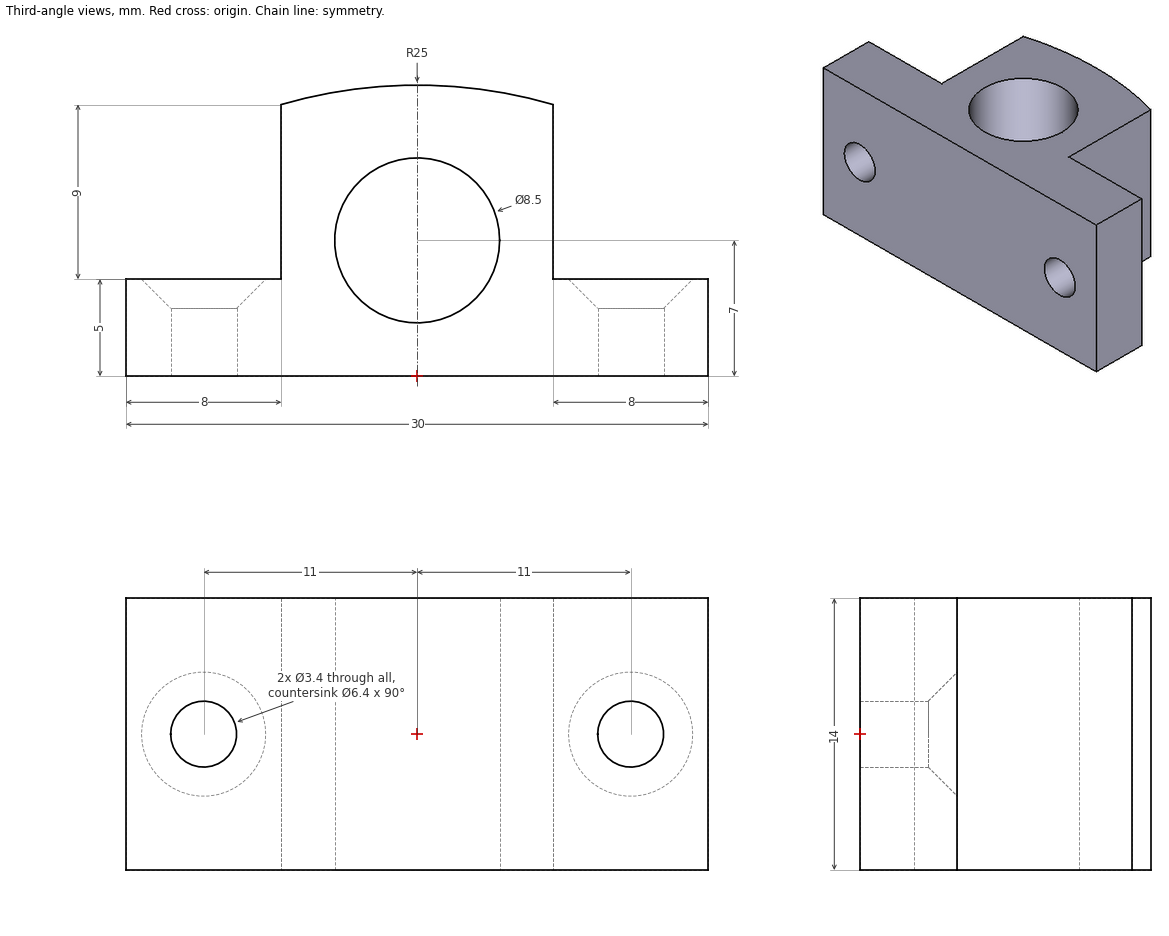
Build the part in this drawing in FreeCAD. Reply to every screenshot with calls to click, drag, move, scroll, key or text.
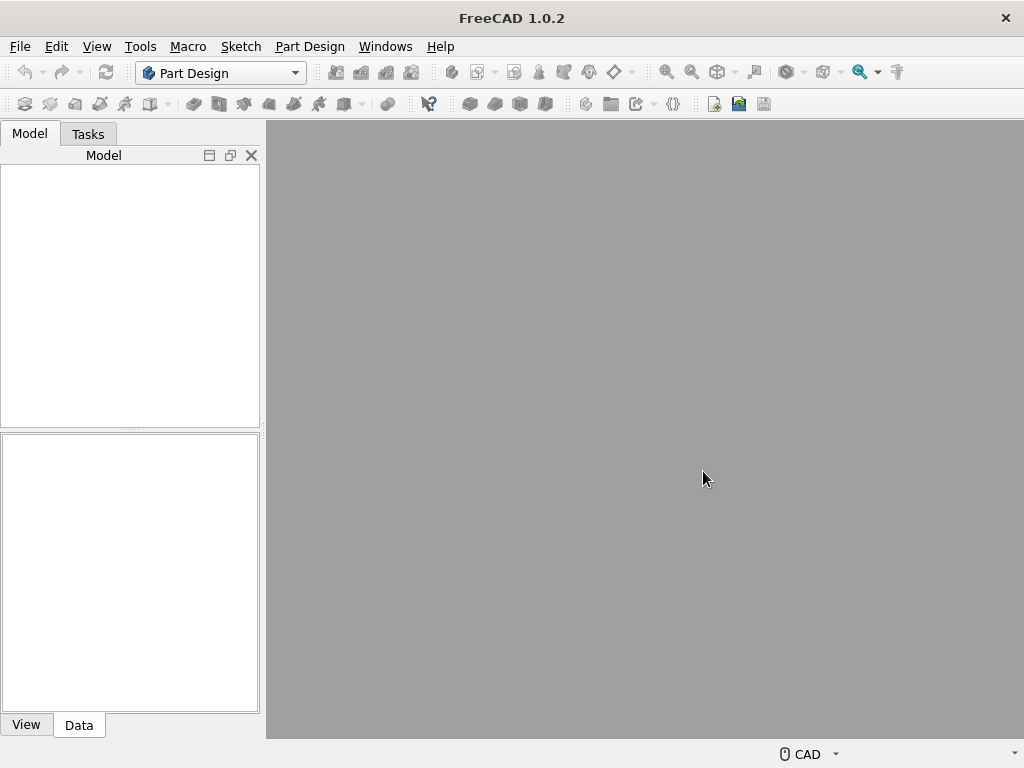
click(714, 104)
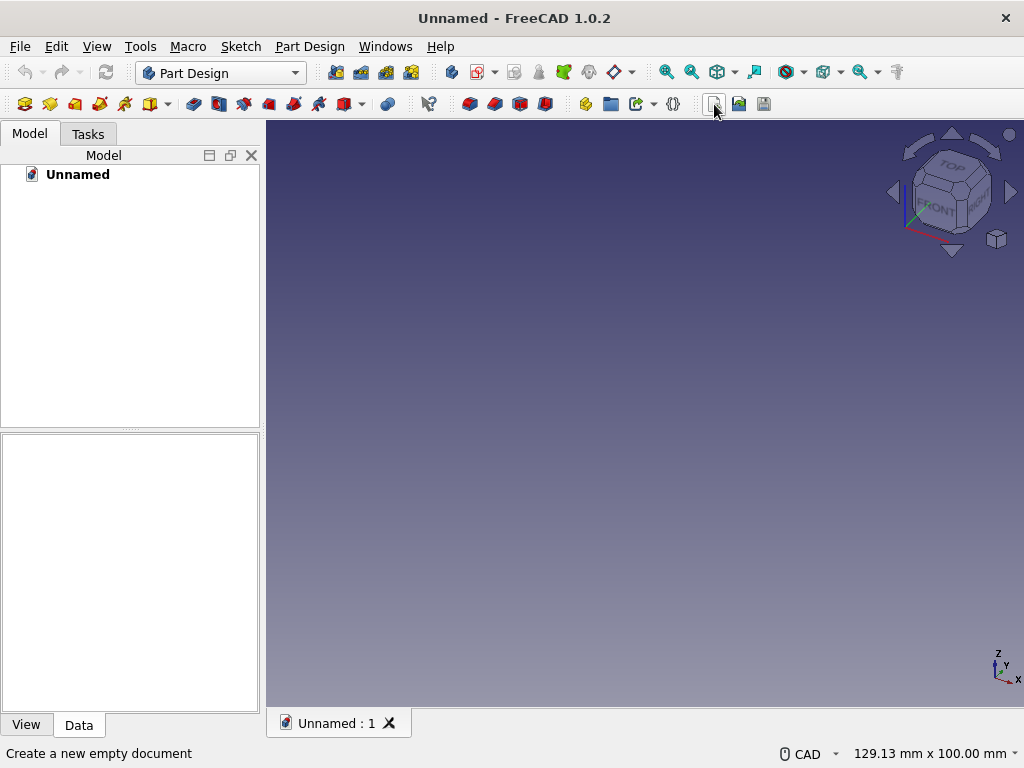
click(476, 72)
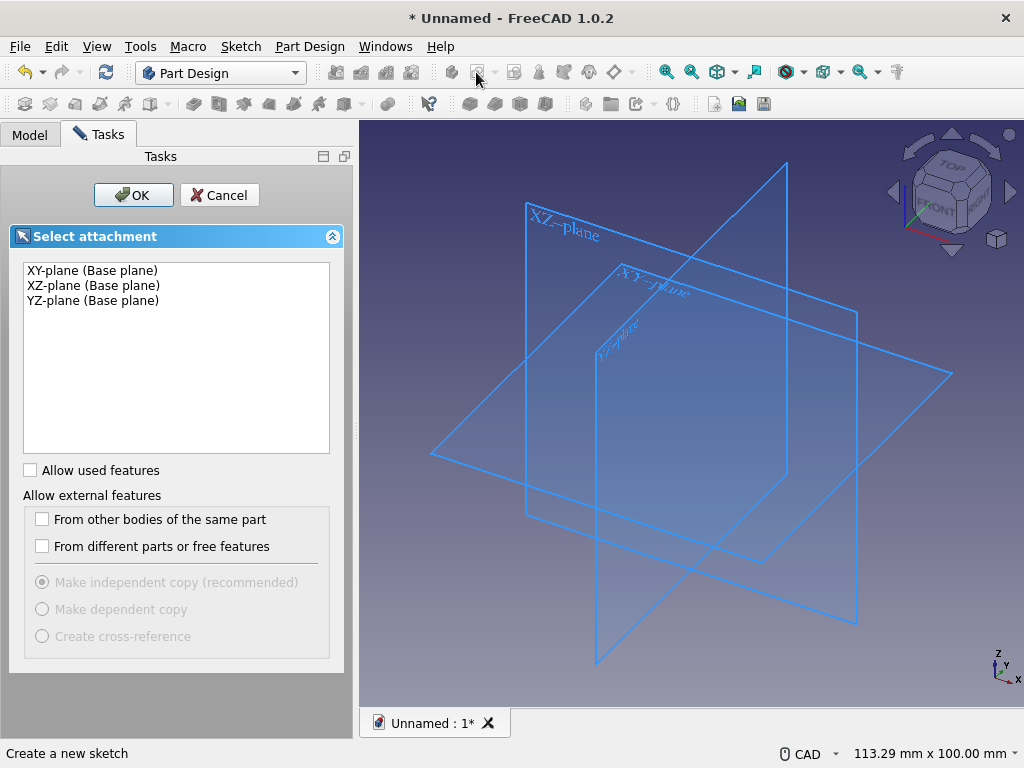
click(84, 270)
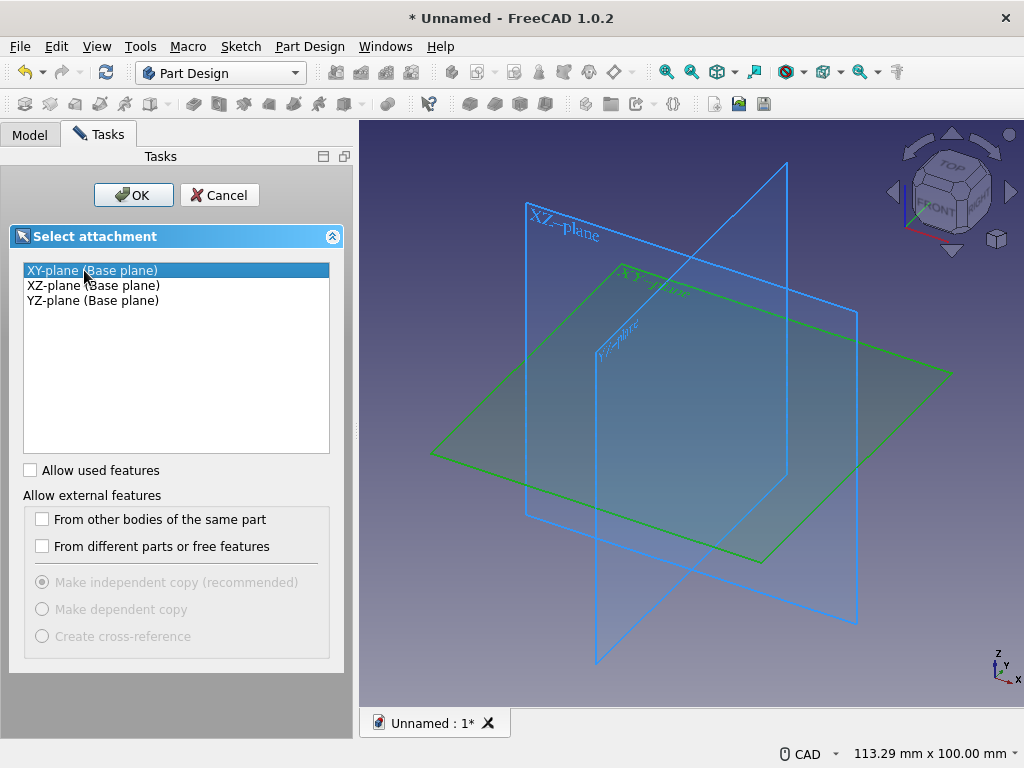
click(134, 195)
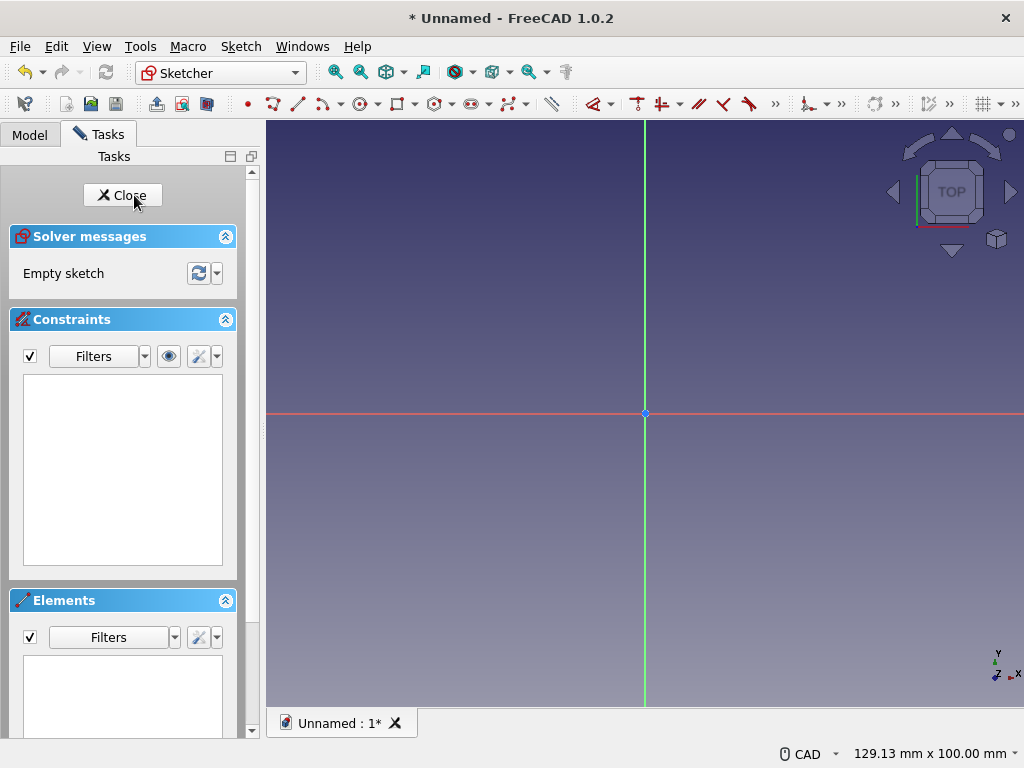
scroll(701, 334, up, 4)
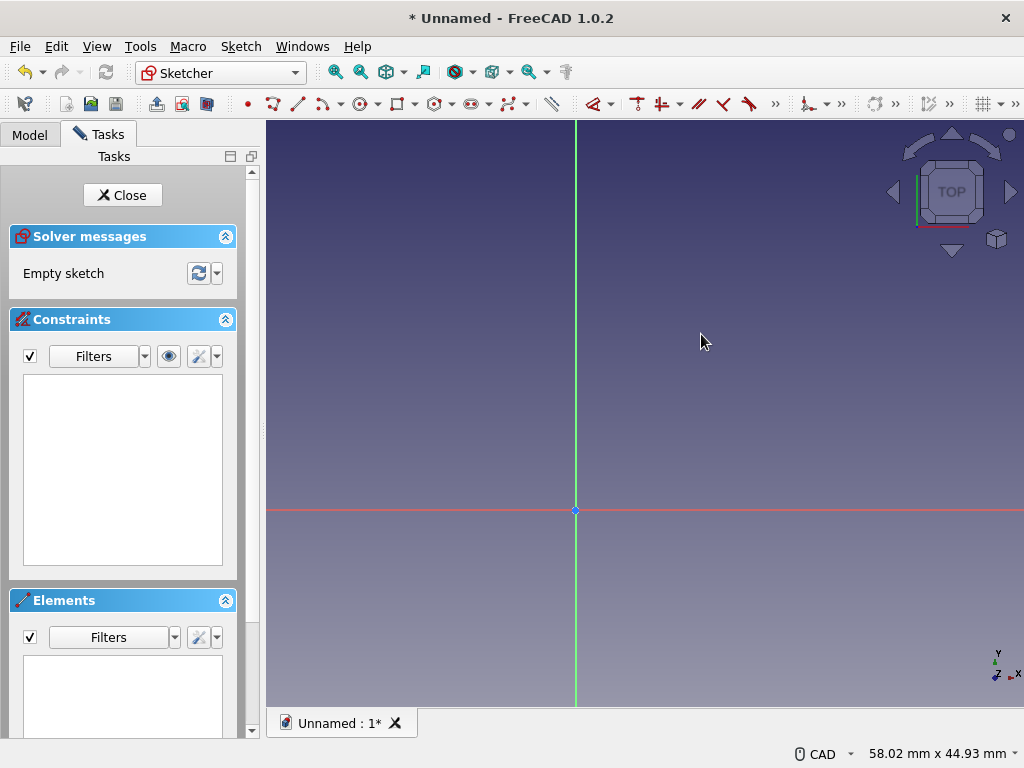
click(273, 104)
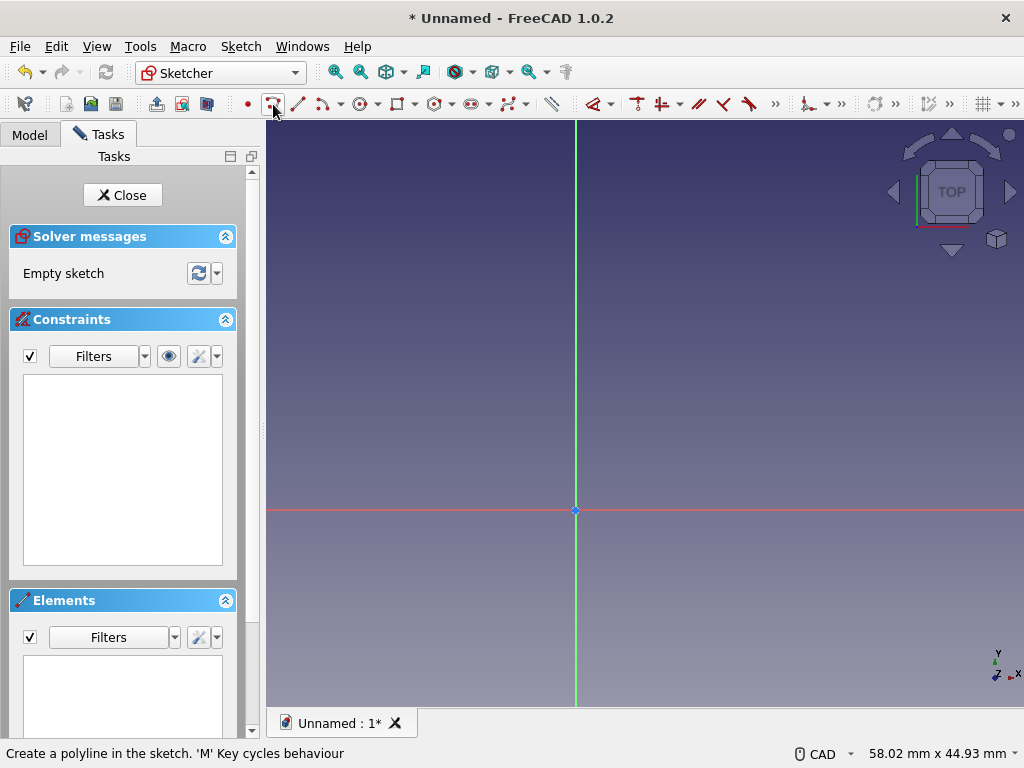
click(484, 328)
click(484, 445)
click(380, 445)
click(380, 510)
click(772, 501)
click(772, 445)
click(667, 445)
click(667, 328)
right_click(667, 328)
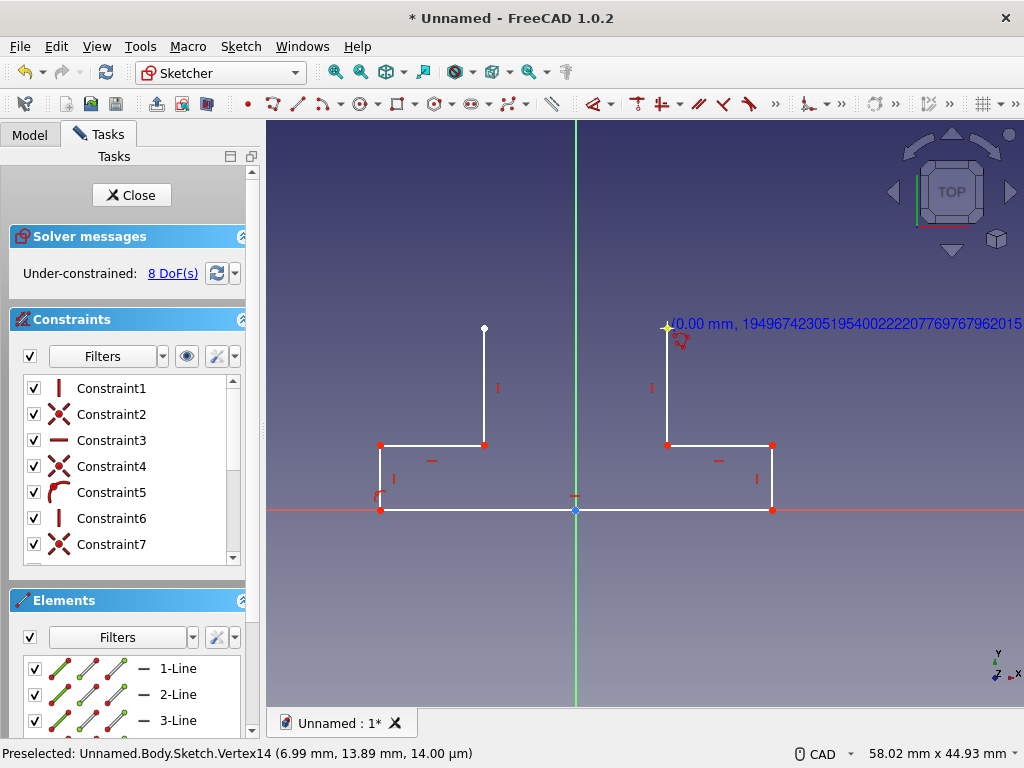
click(340, 104)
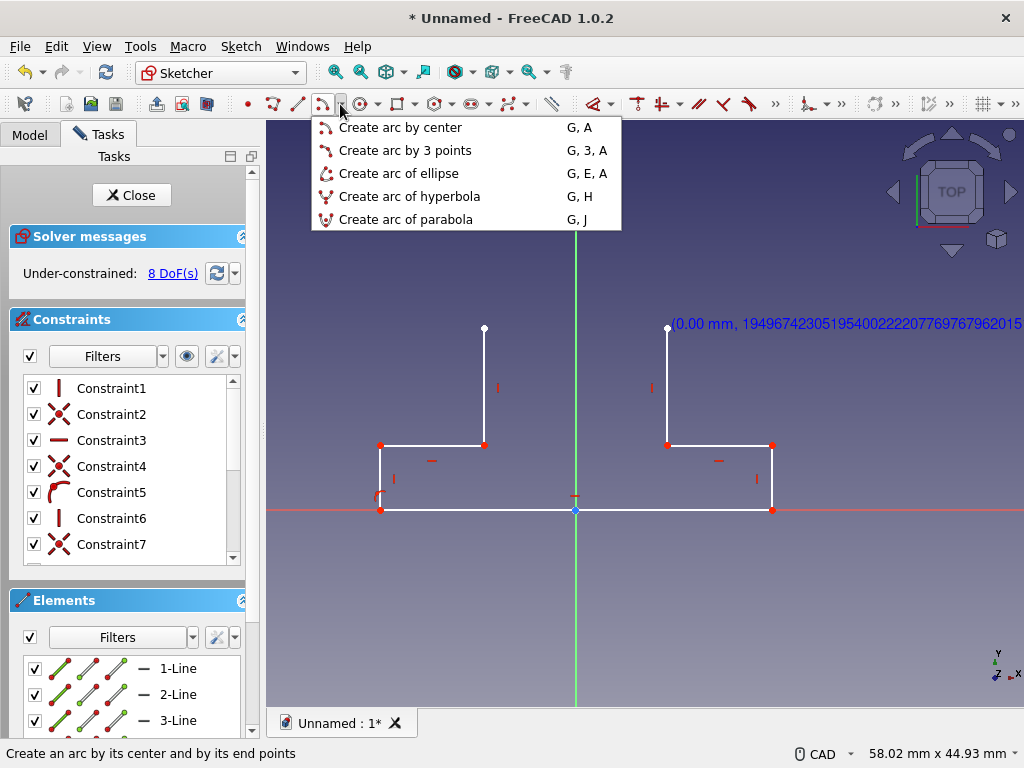
click(466, 150)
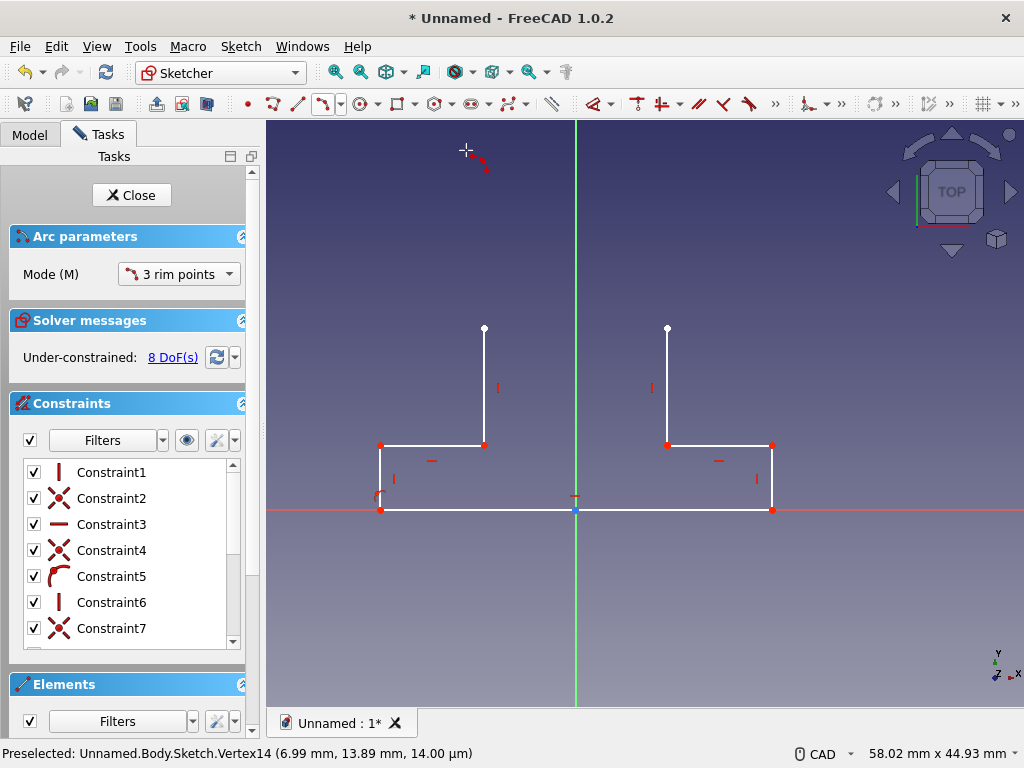
click(667, 329)
click(484, 329)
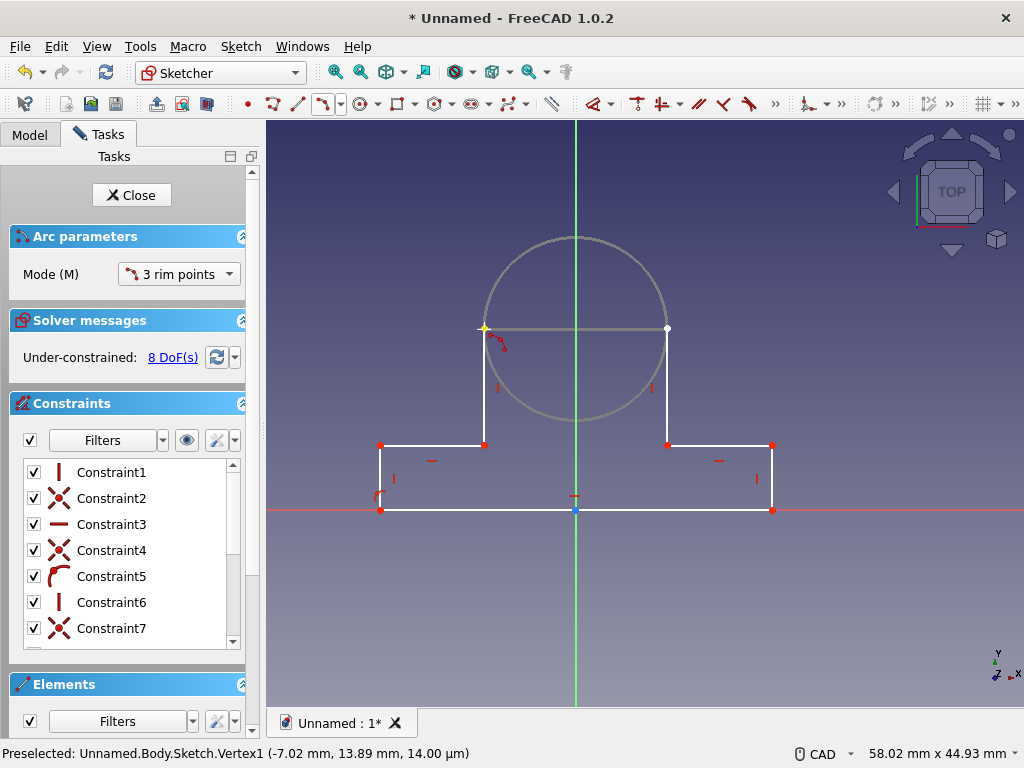
scroll(594, 315, up, 2)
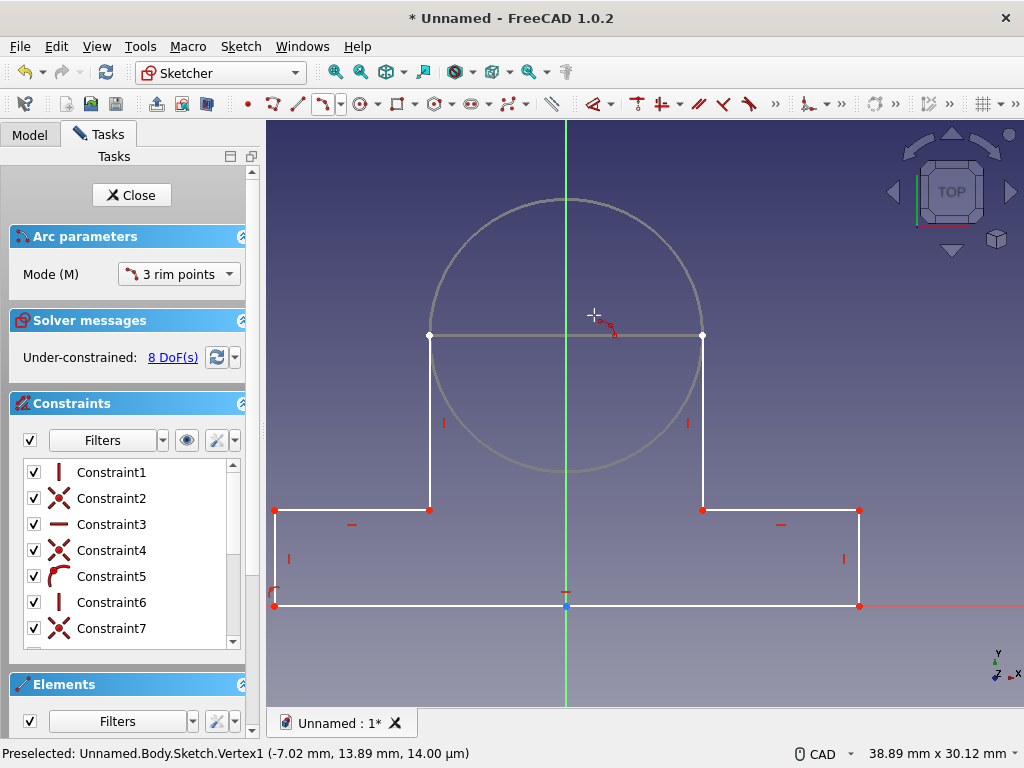
click(594, 315)
key(Escape)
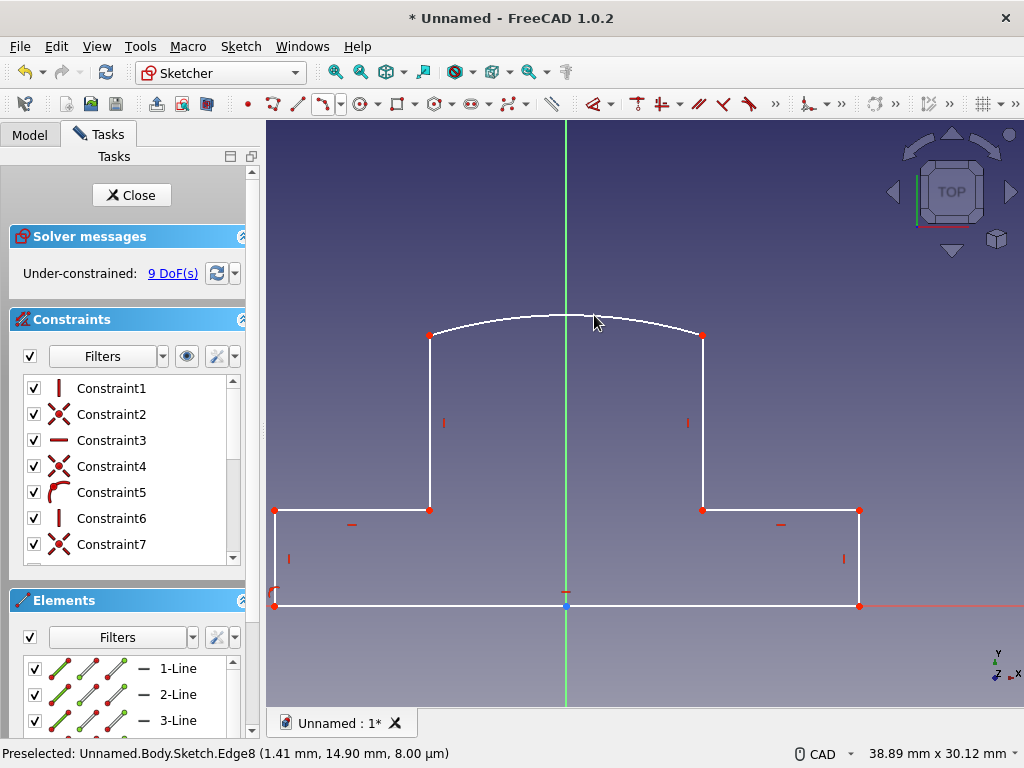
scroll(597, 318, down, 2)